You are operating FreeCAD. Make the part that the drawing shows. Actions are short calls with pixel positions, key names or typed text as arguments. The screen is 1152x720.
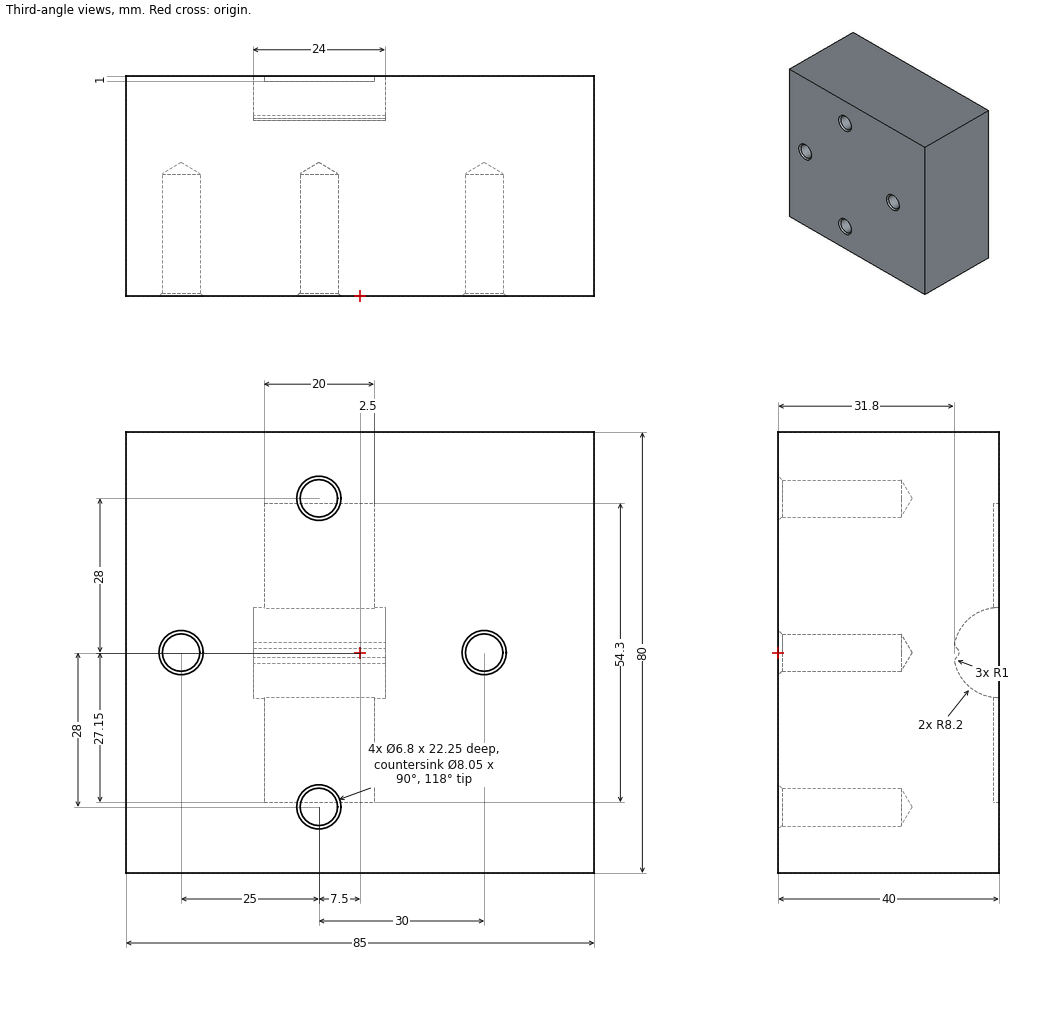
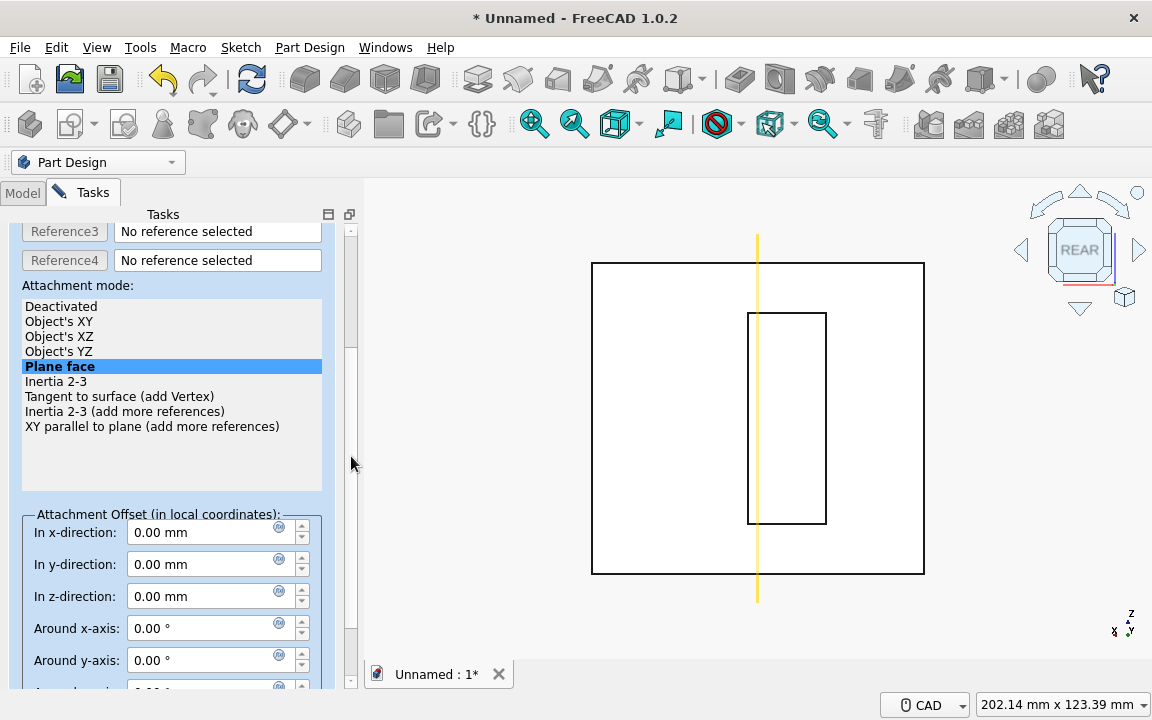
triple_click(210, 596)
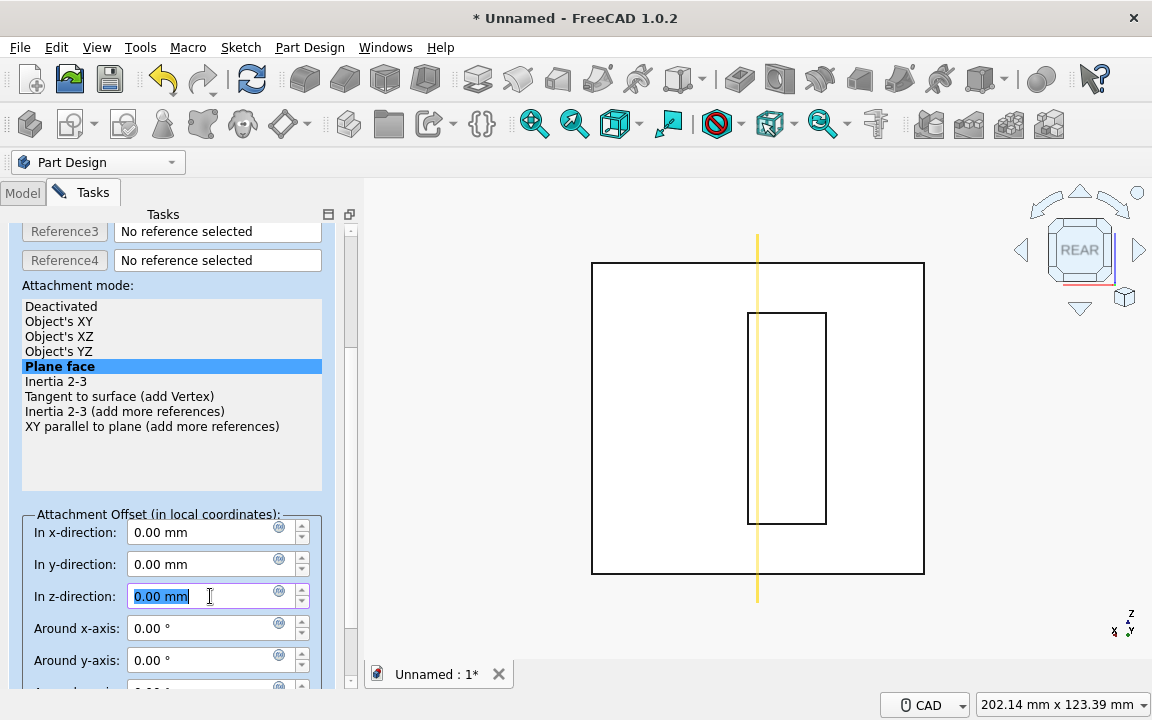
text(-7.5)
key(Tab)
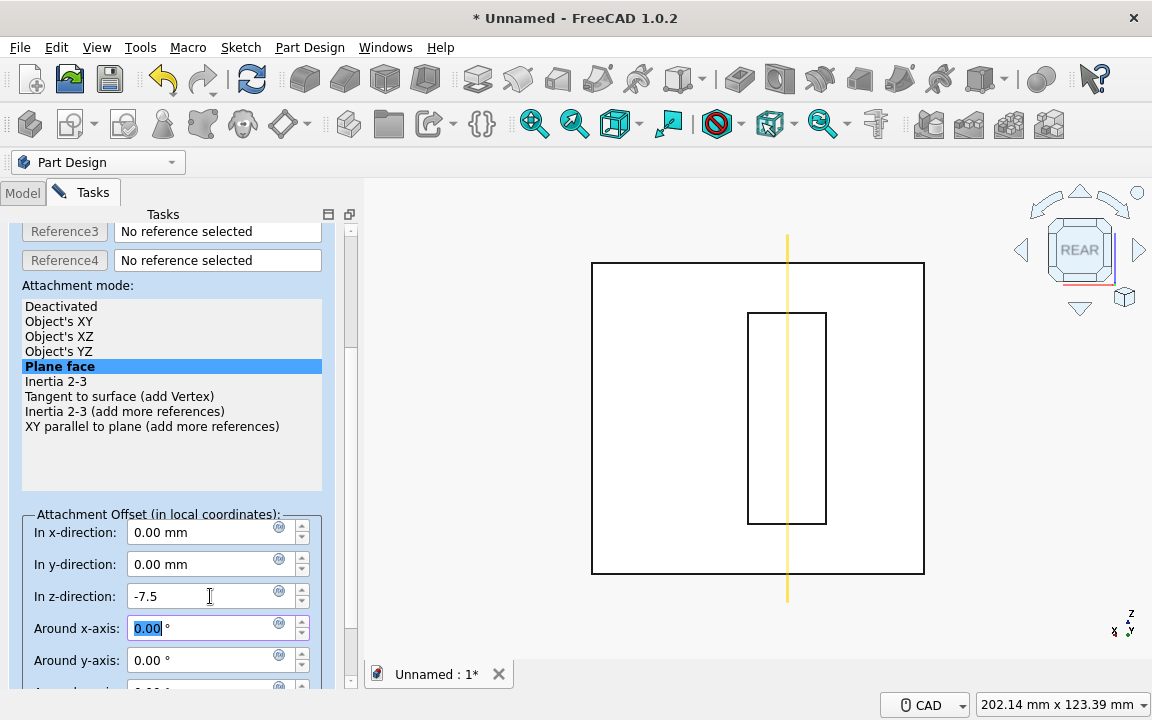
scroll(351, 456, up, 4)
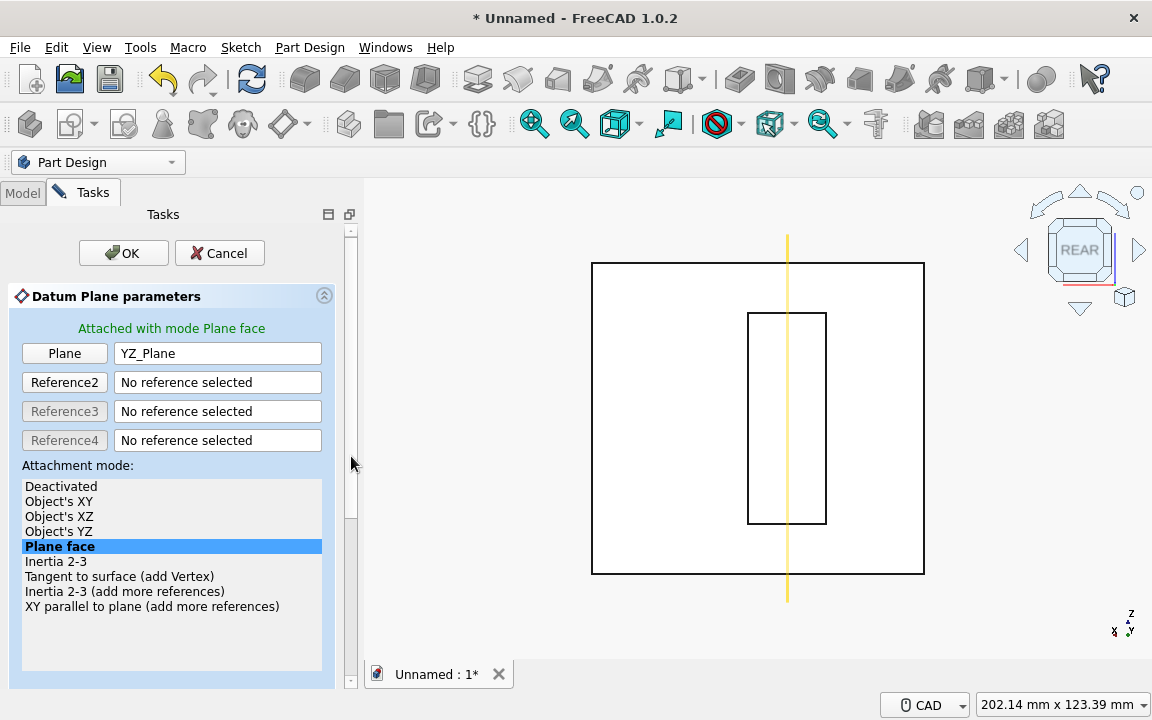
click(124, 253)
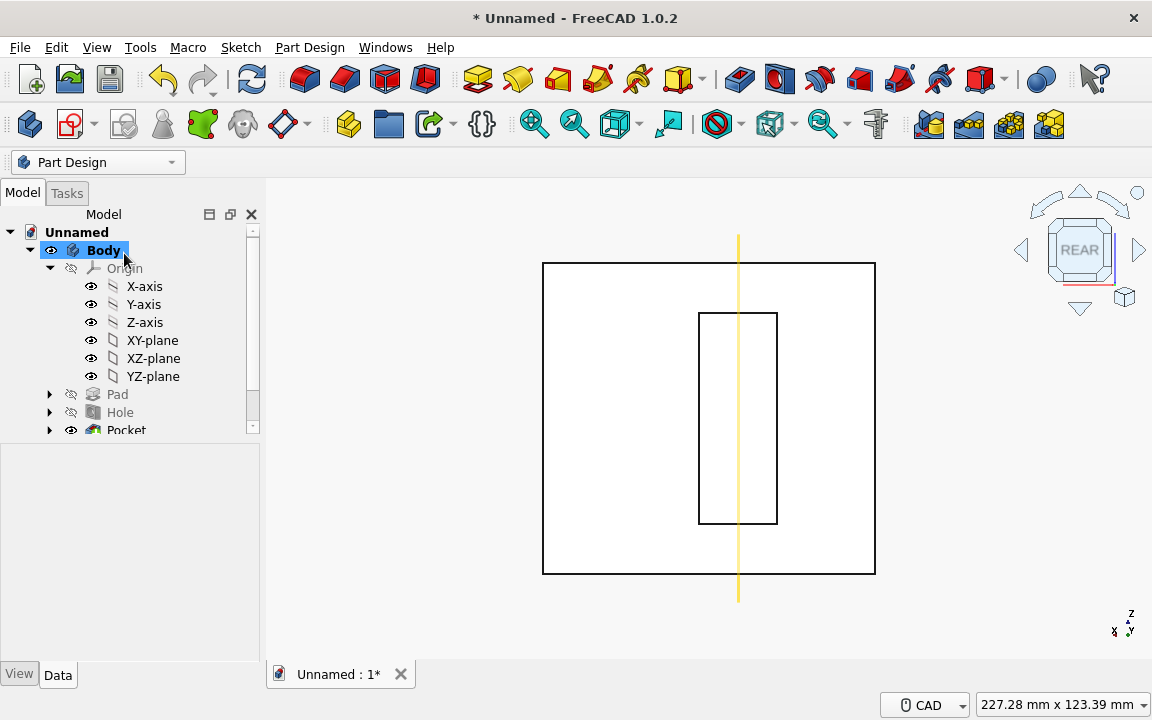
scroll(100, 336, down, 3)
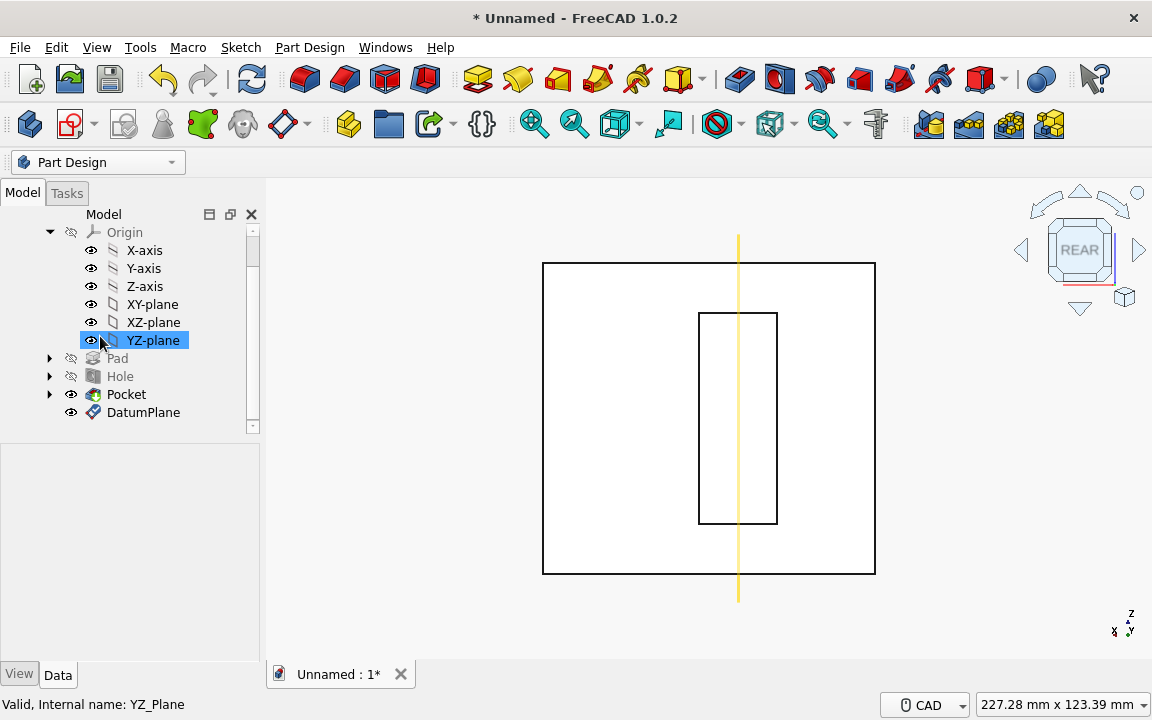
click(116, 412)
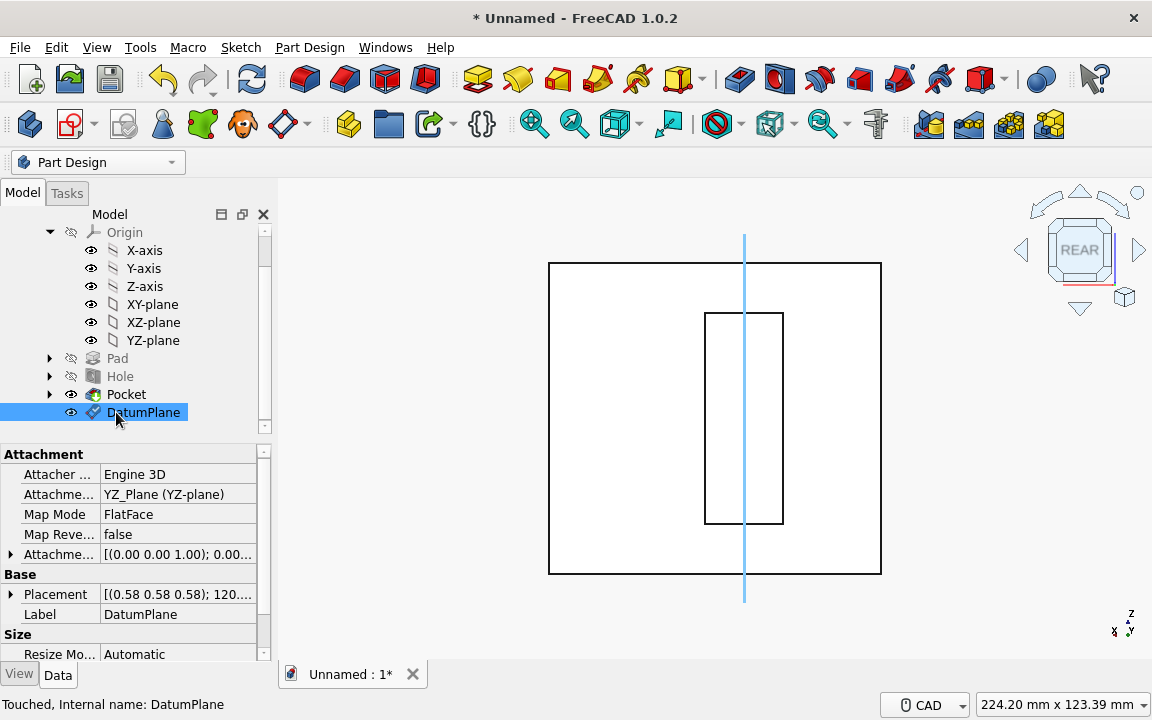
click(70, 124)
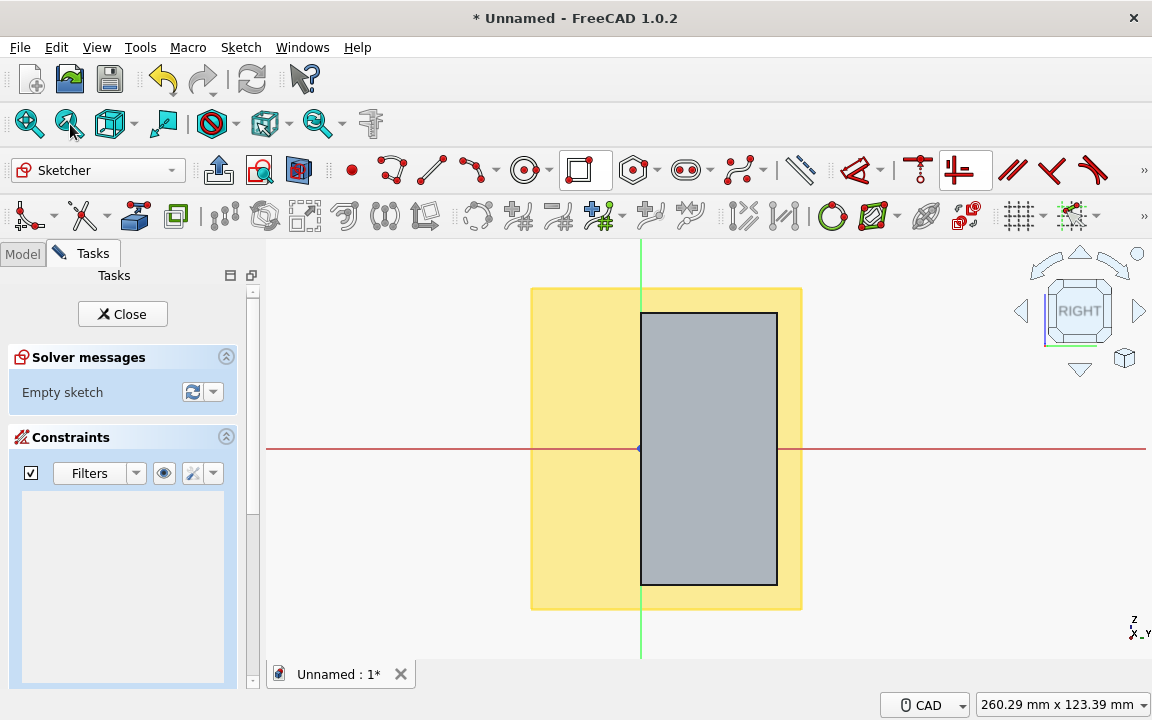
click(300, 170)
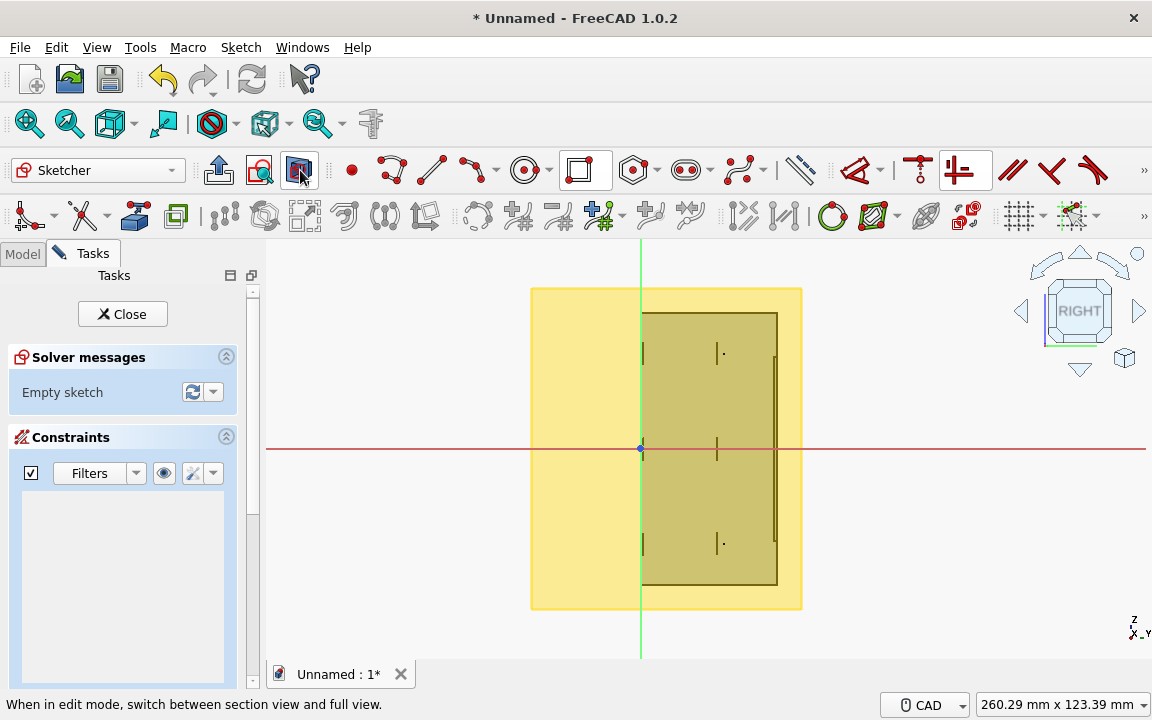
scroll(739, 449, up, 6)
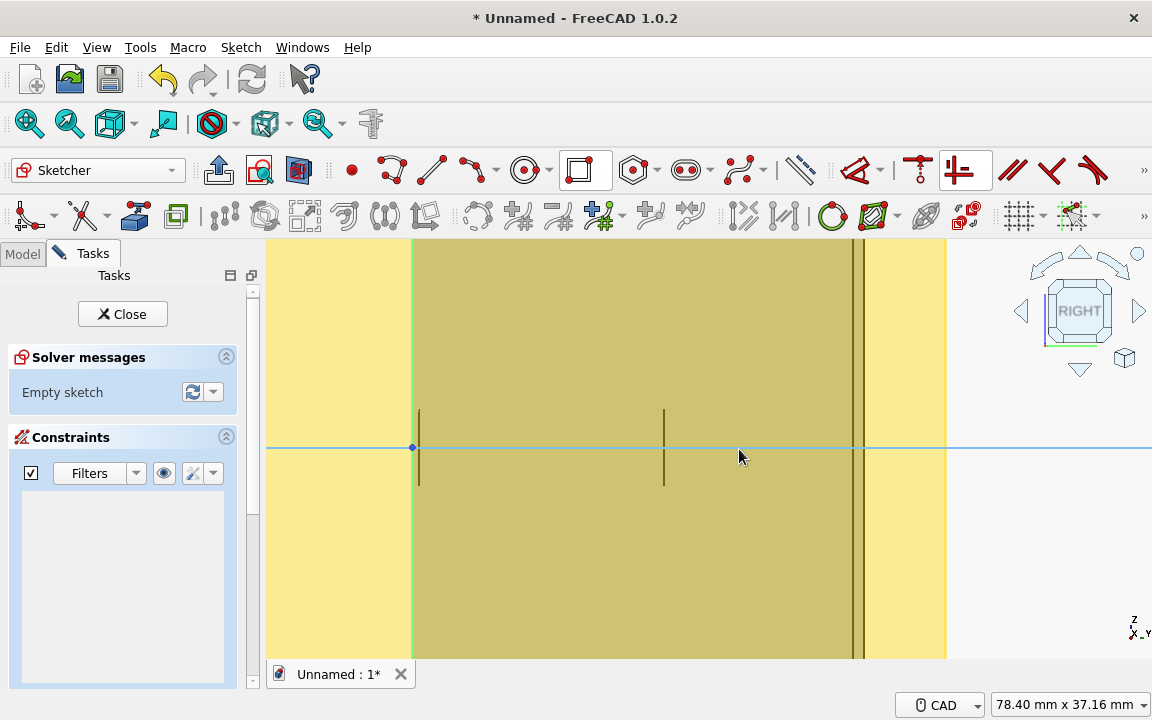
click(432, 170)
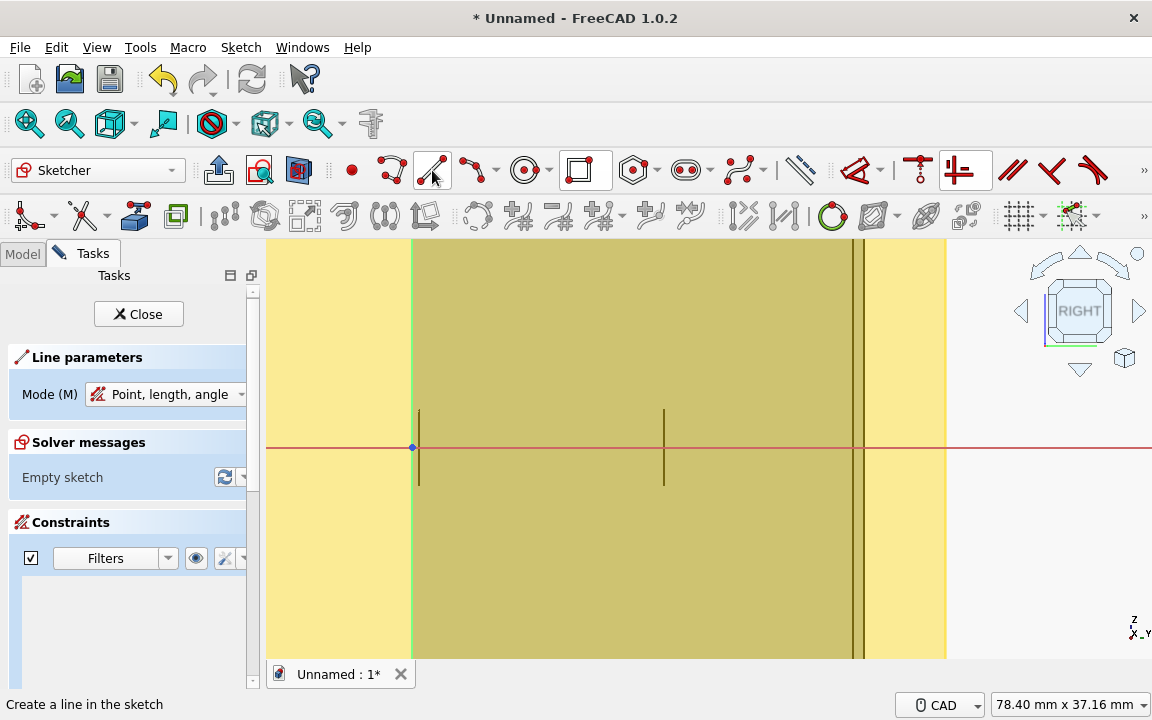
click(864, 355)
click(864, 541)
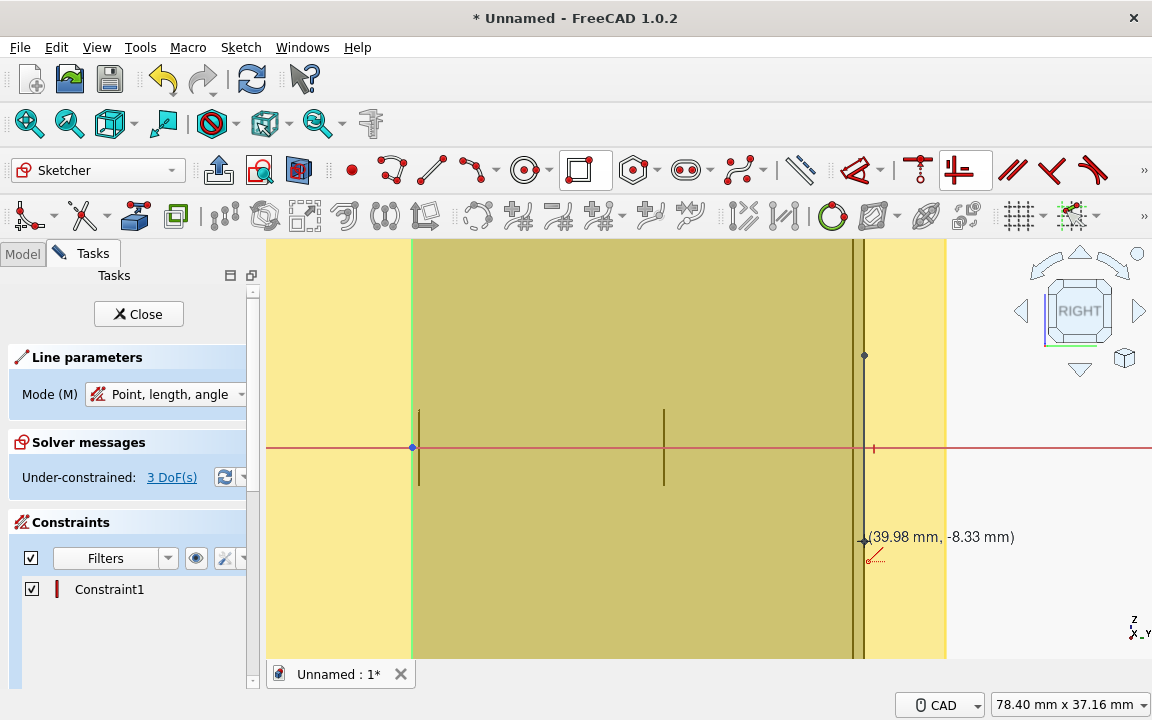
click(472, 170)